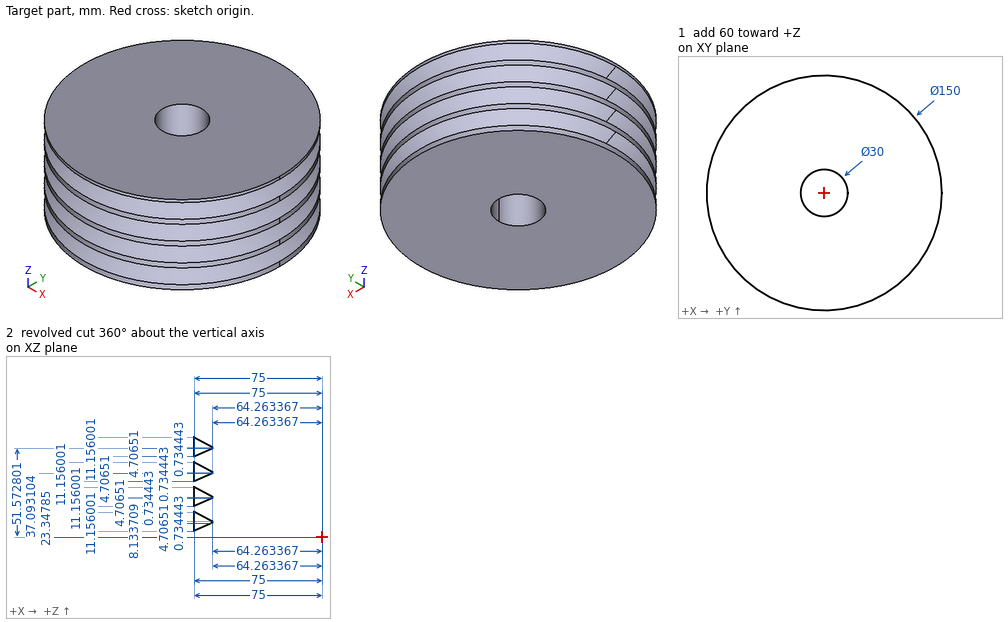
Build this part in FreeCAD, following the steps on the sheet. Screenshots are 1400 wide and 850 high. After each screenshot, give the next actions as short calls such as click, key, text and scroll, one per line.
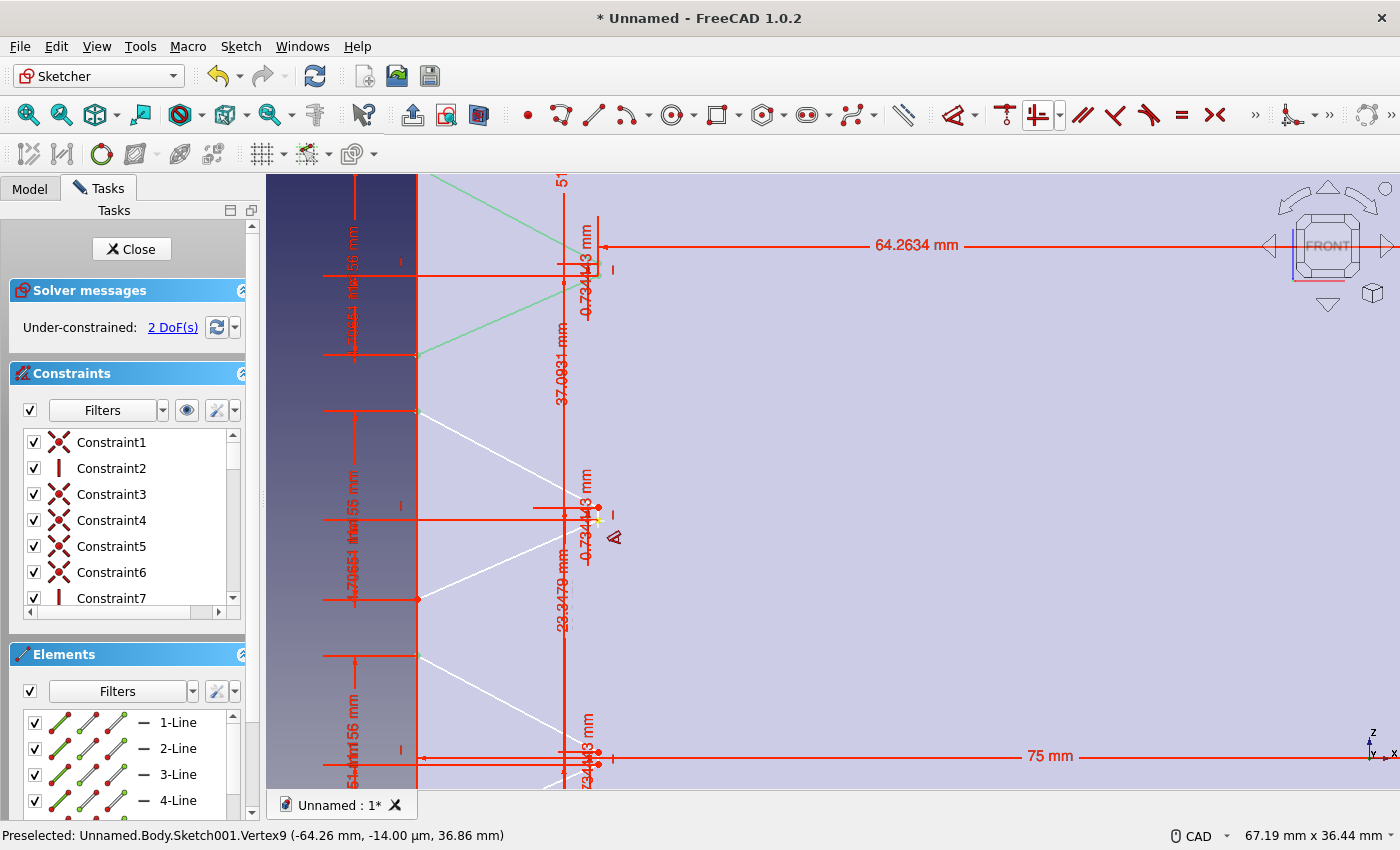
click(598, 520)
click(917, 486)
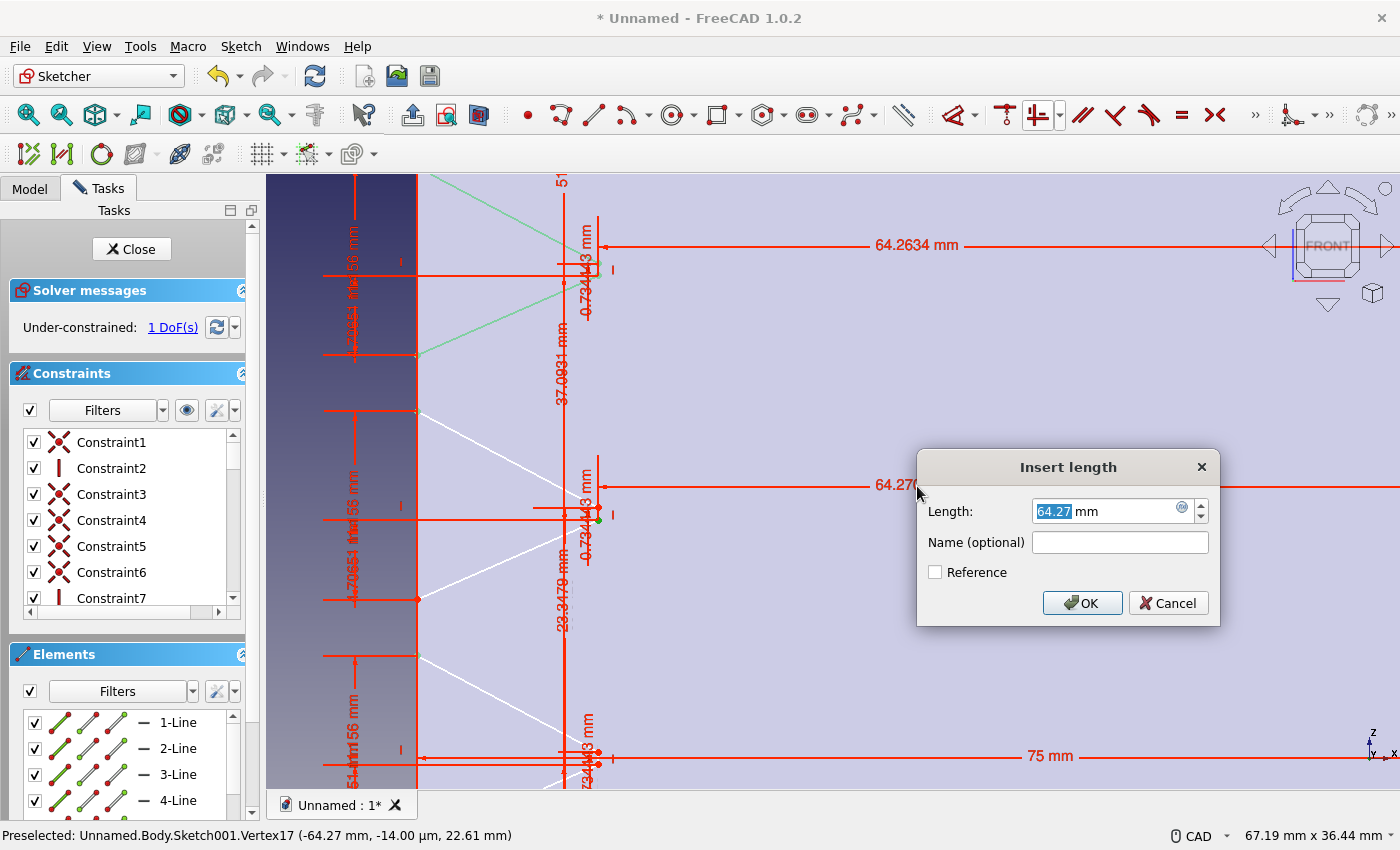
text(64.263367)
key(Return)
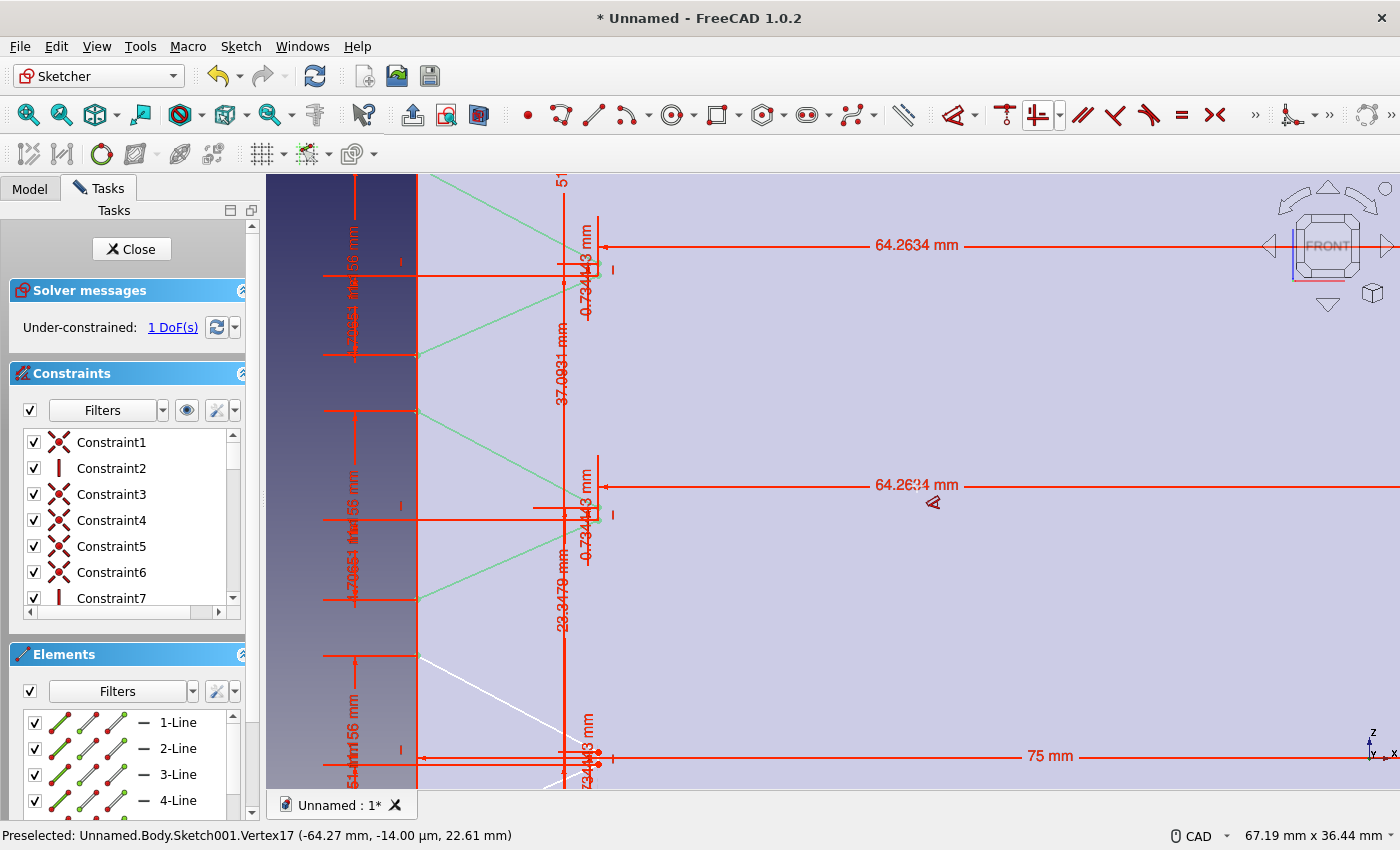
scroll(598, 522, down, 5)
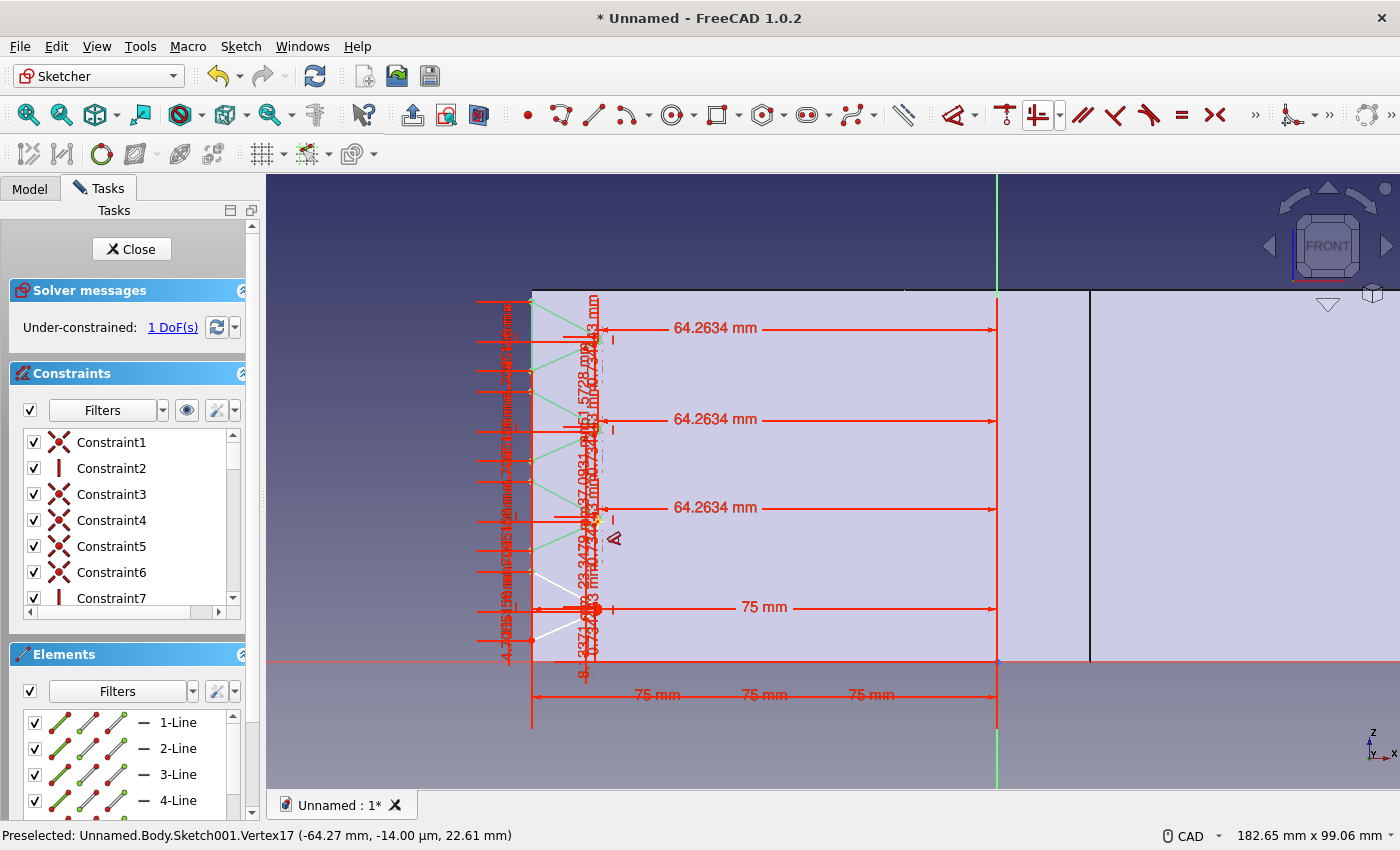
scroll(598, 612, up, 5)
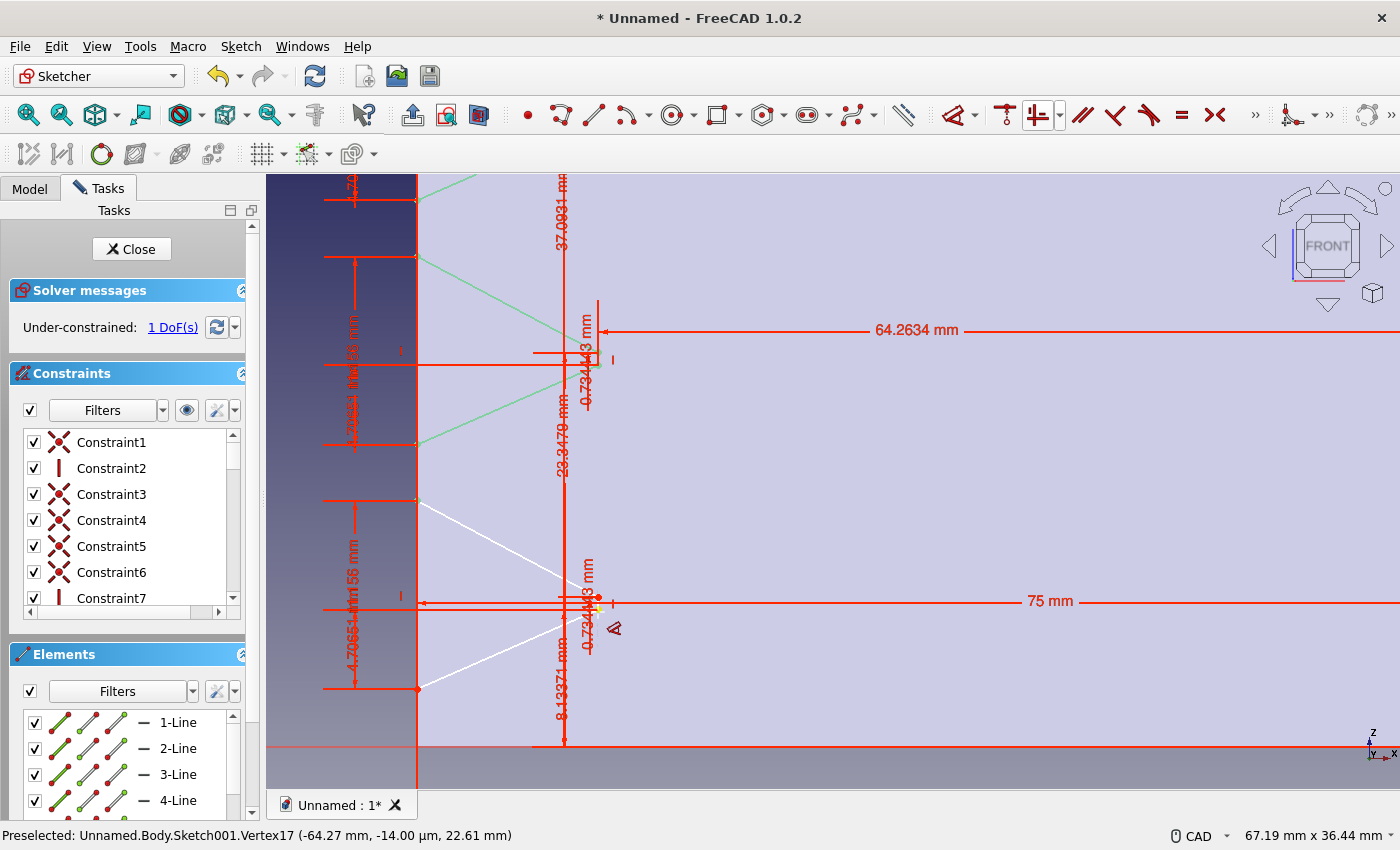
click(598, 610)
click(917, 576)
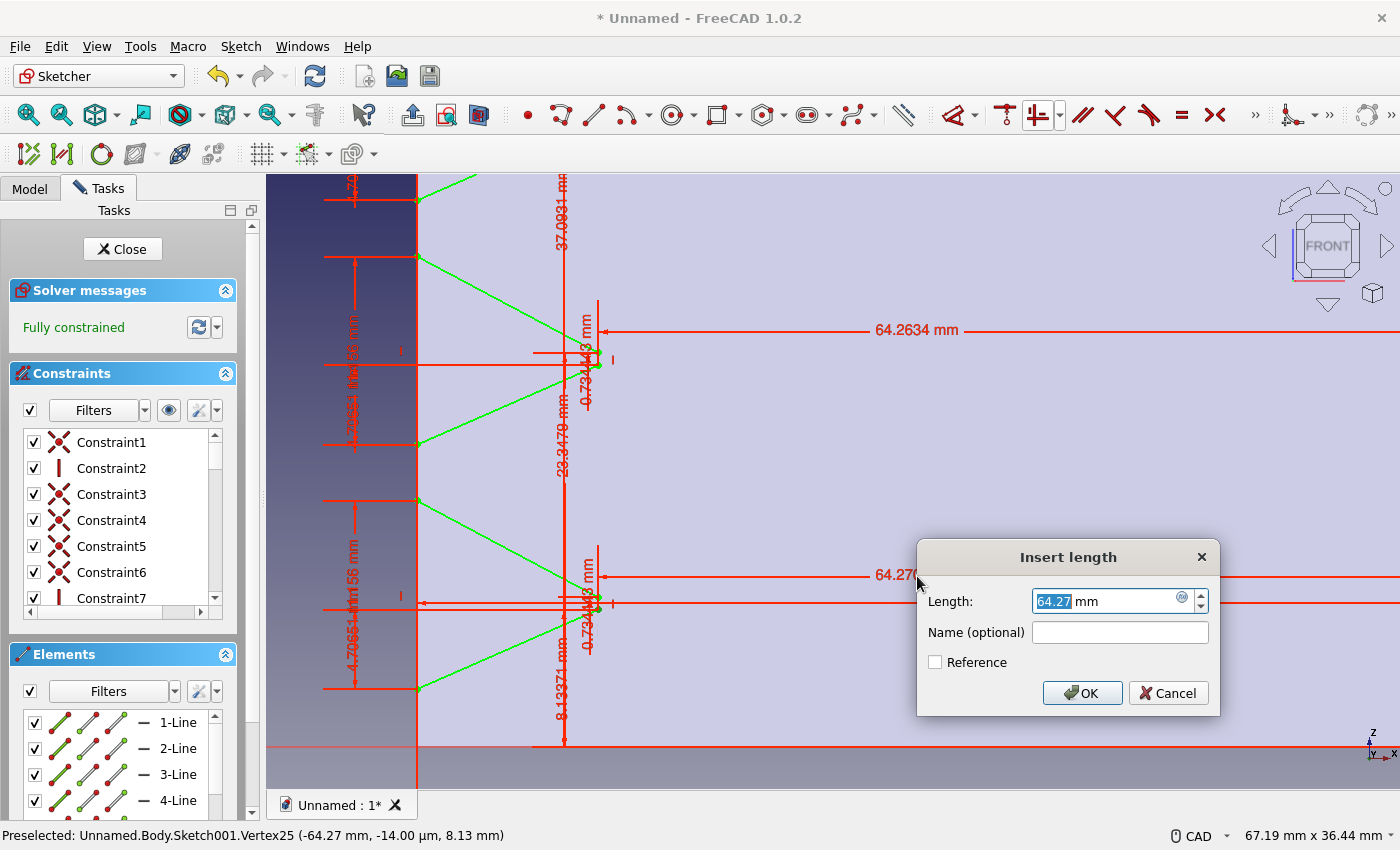
text(64.263367)
key(Return)
key(Escape)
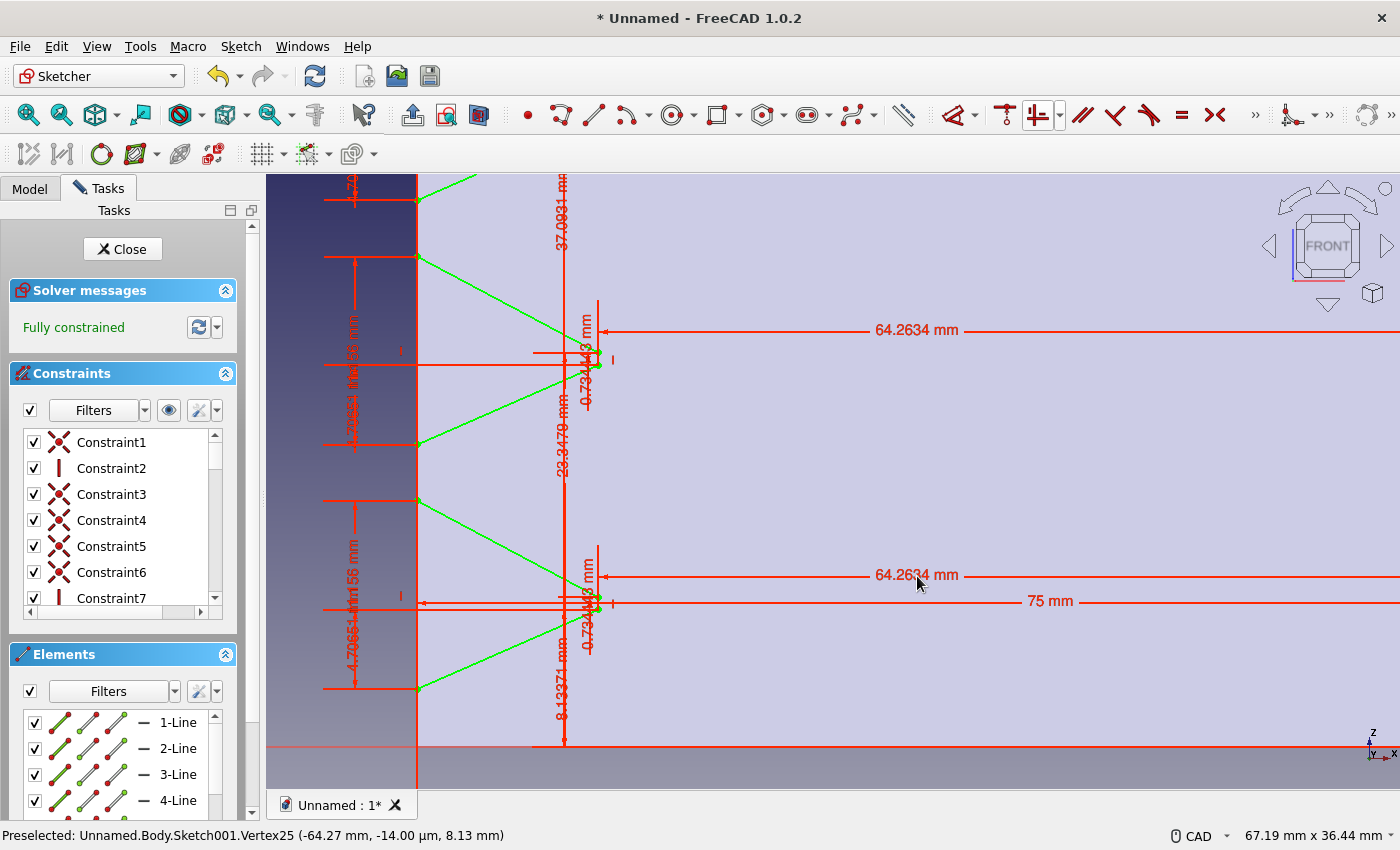
click(123, 249)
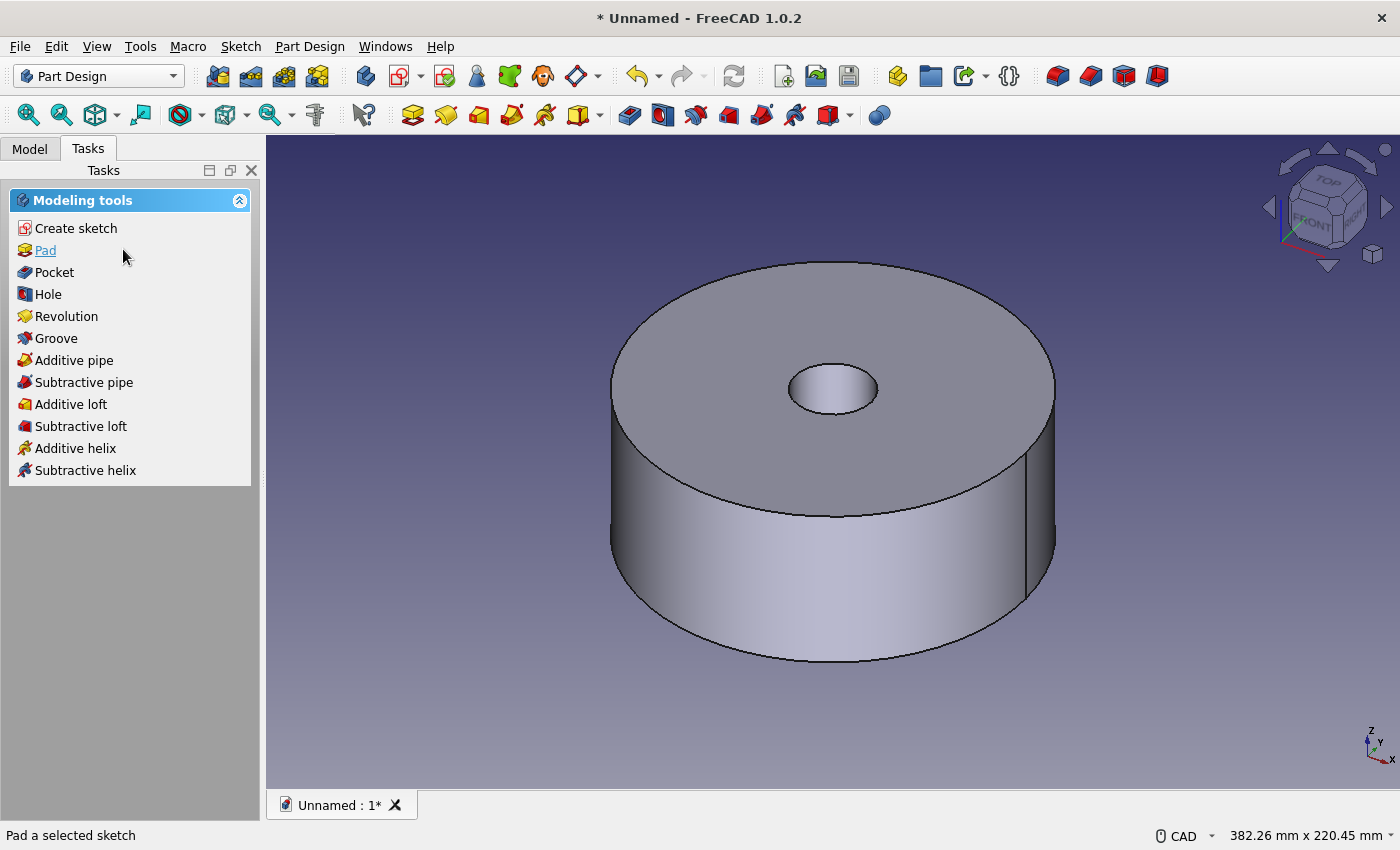
click(696, 116)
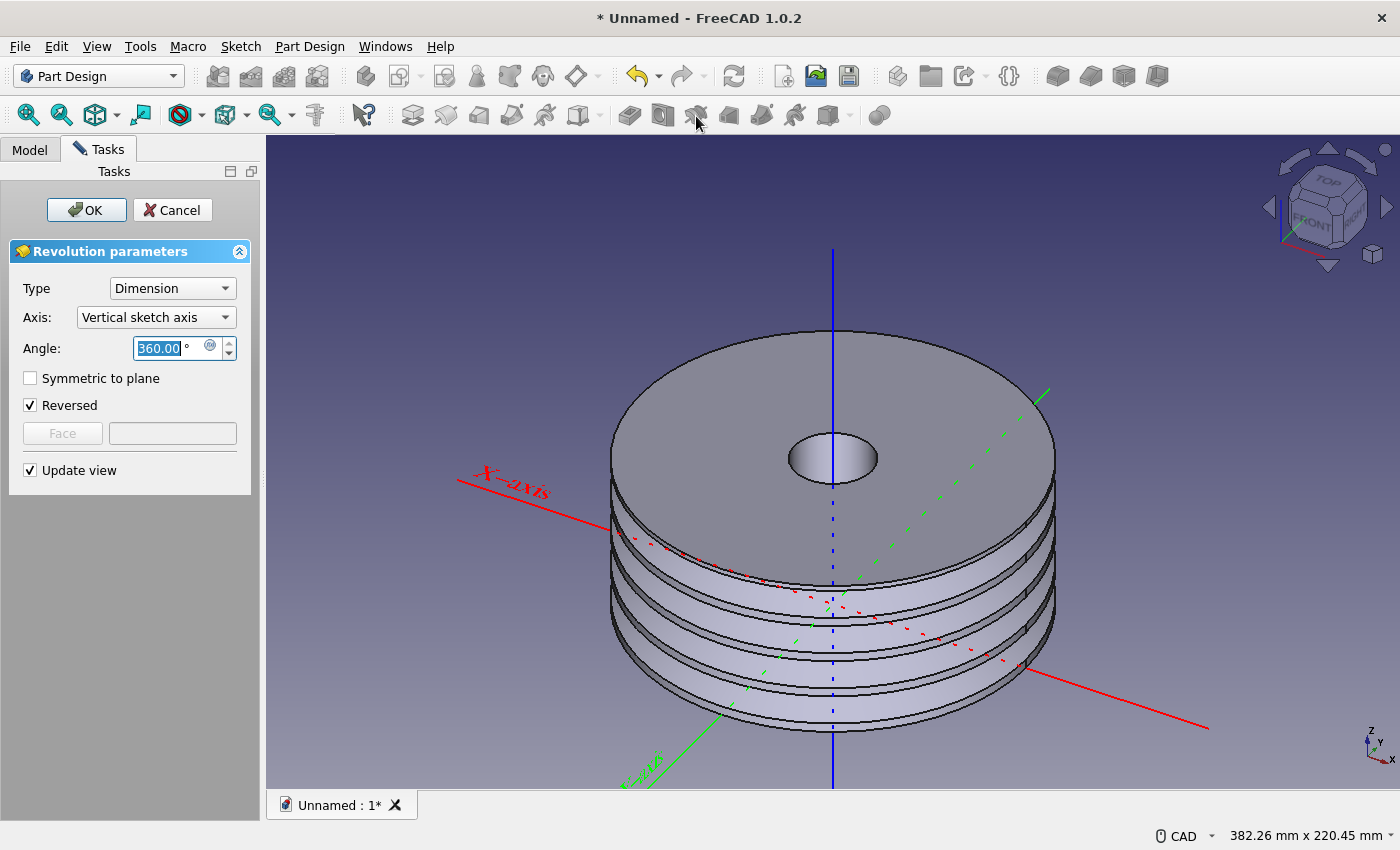
click(87, 210)